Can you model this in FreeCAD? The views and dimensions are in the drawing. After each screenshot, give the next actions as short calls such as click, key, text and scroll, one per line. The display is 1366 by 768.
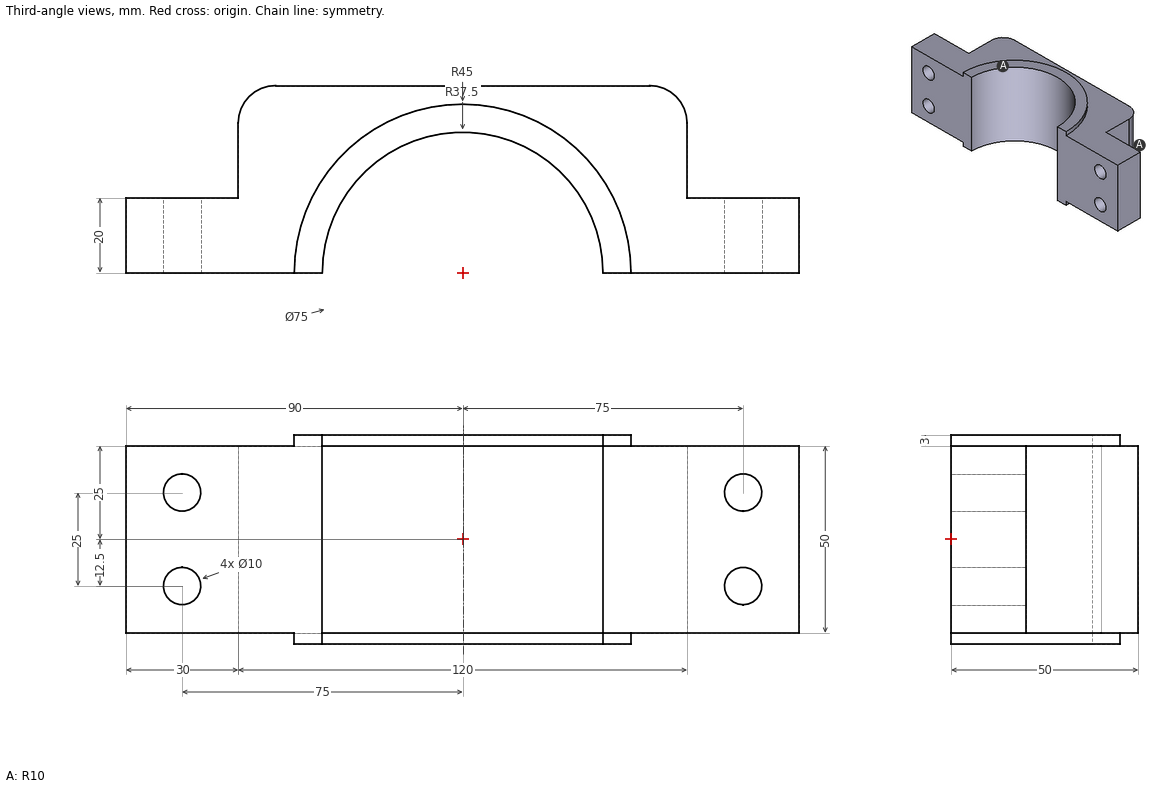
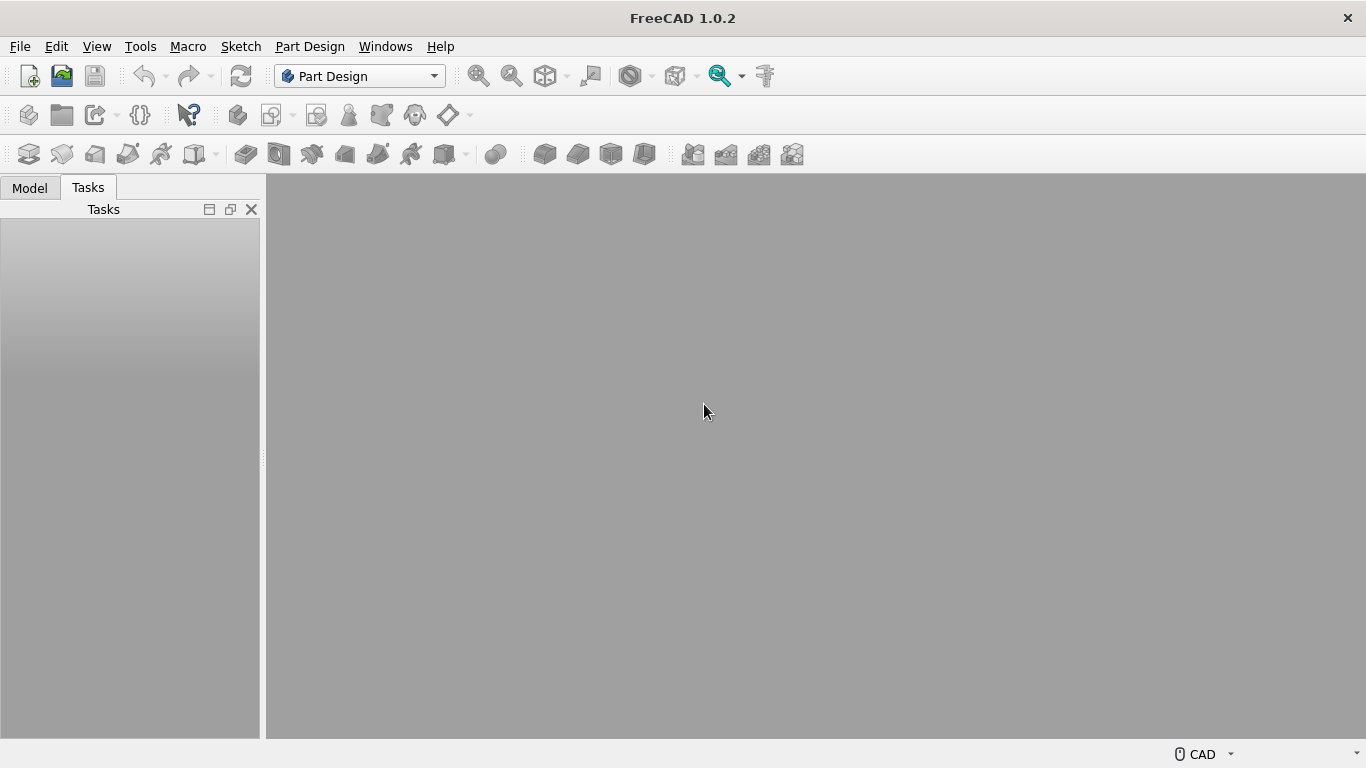
click(29, 76)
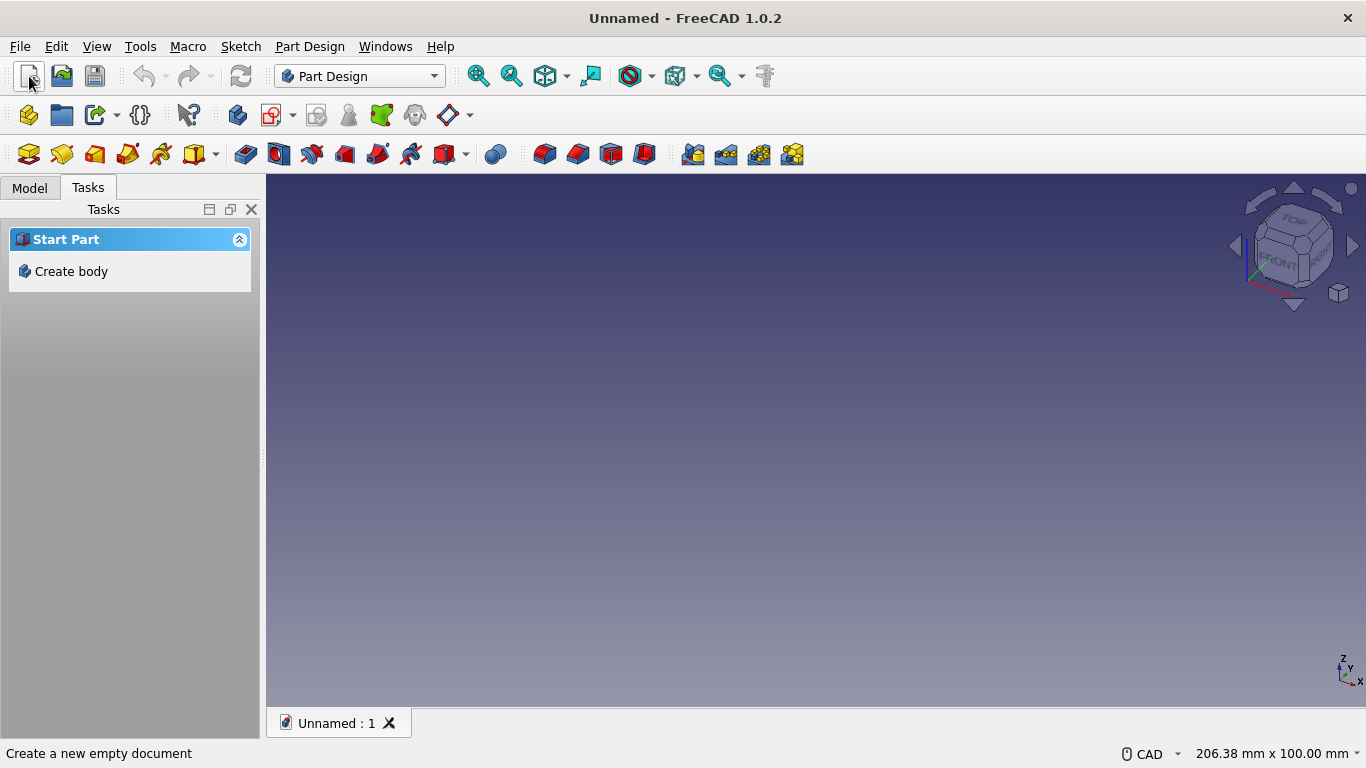
click(270, 116)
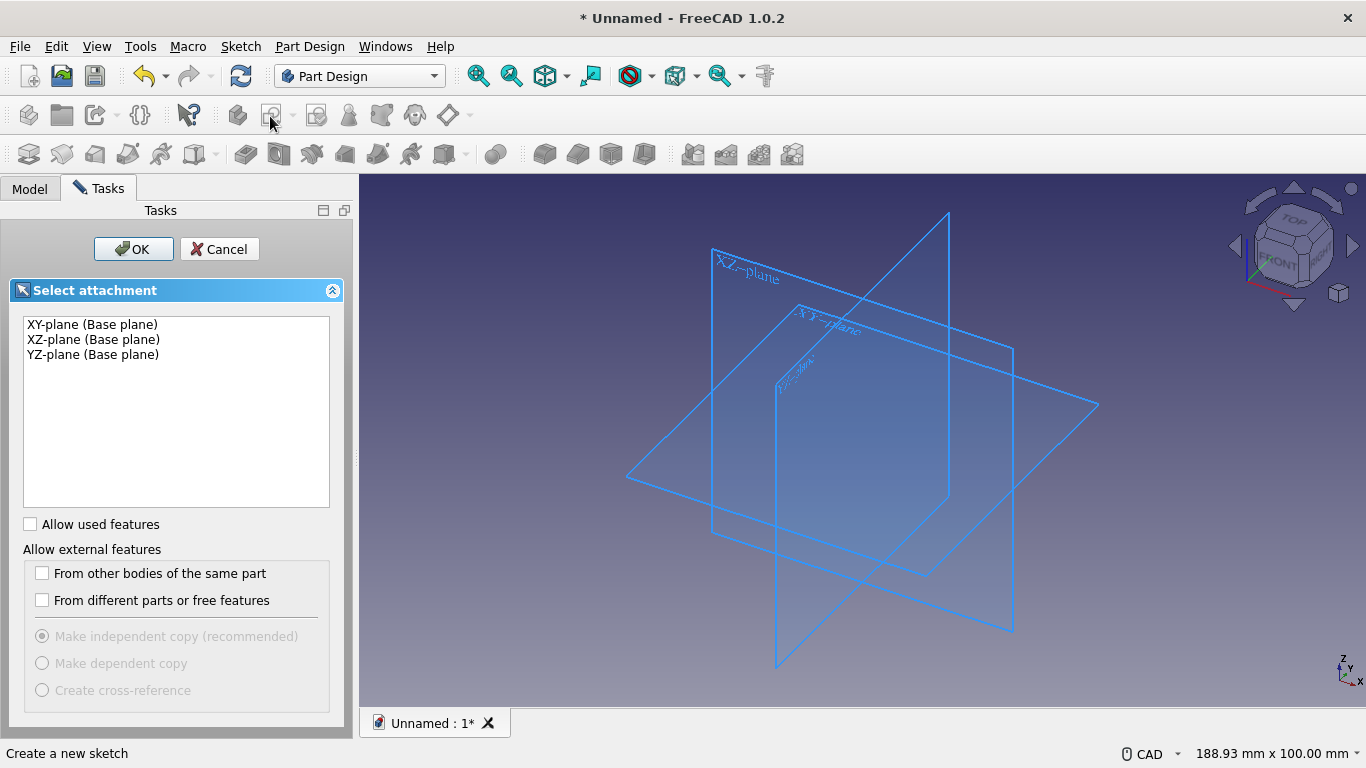
click(84, 340)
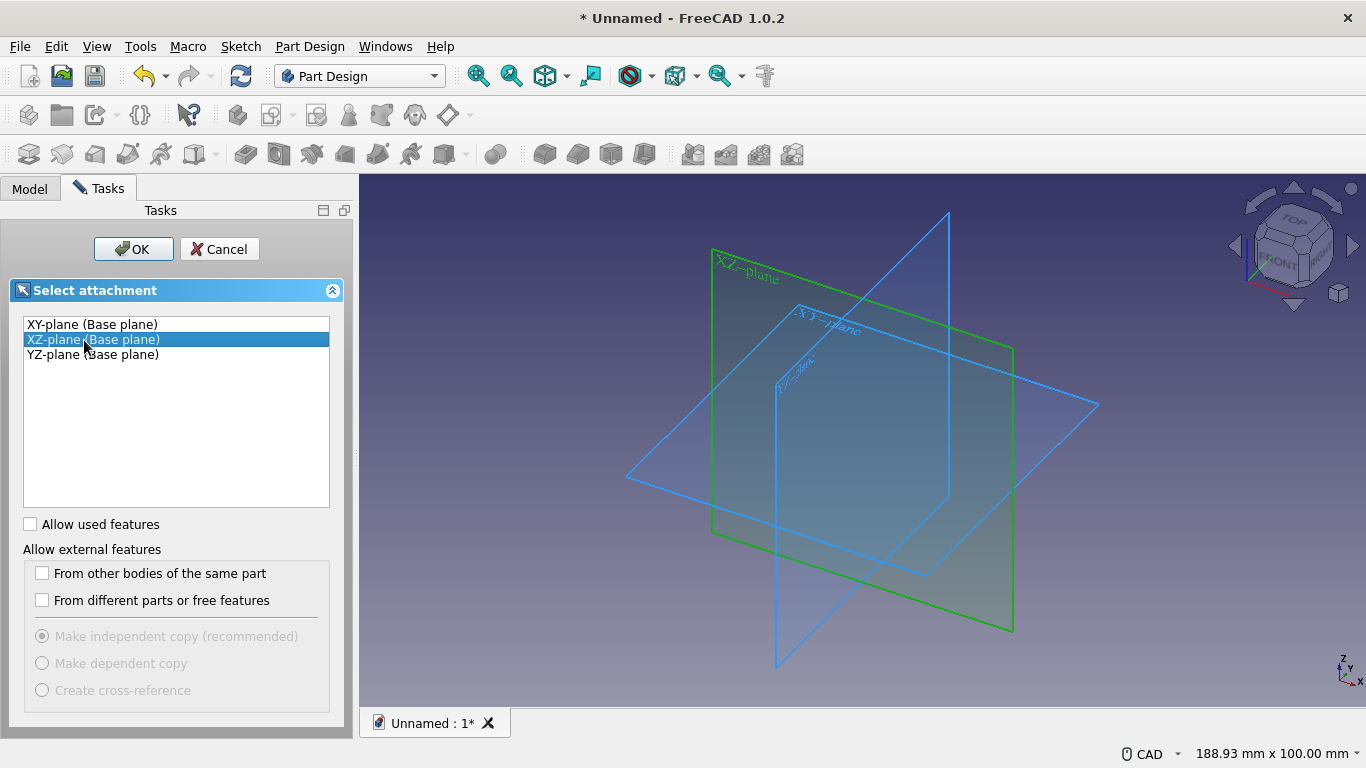
click(134, 249)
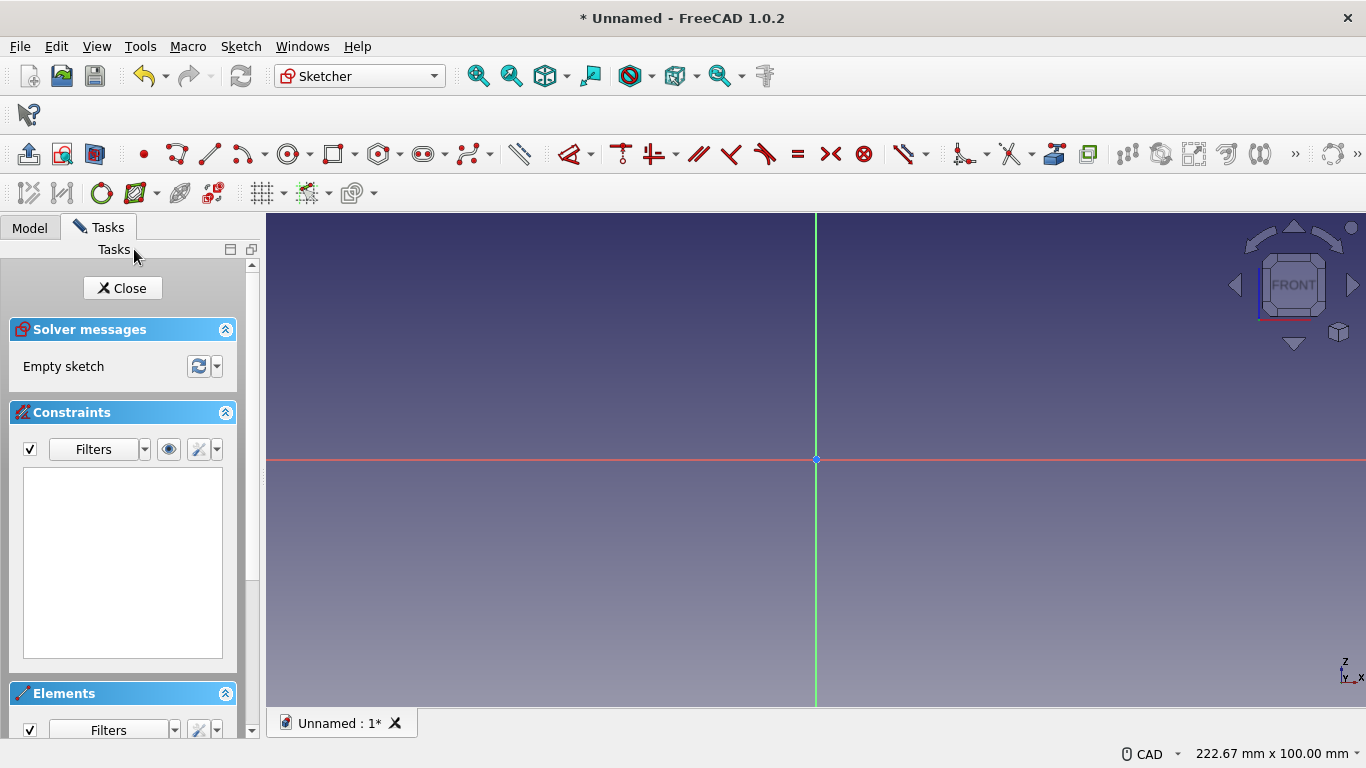
key(g)
key(v)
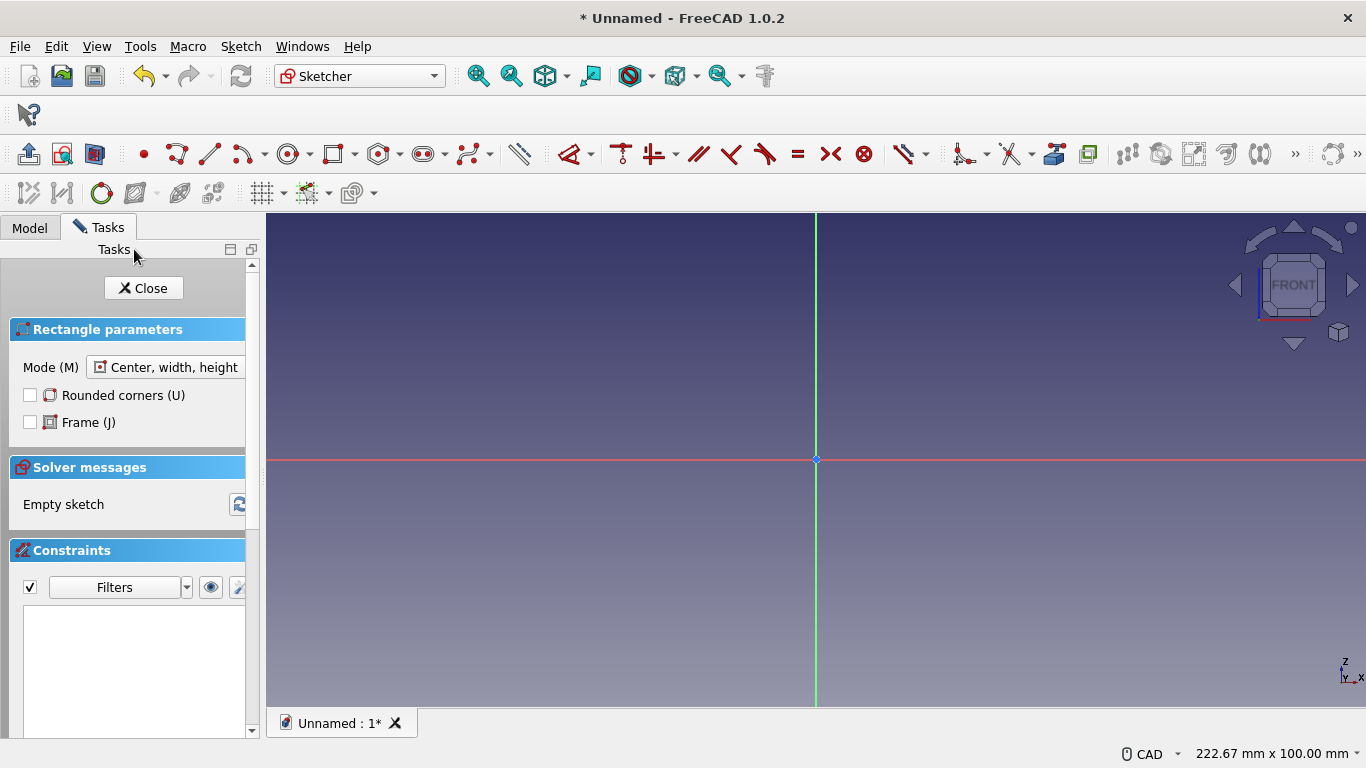
click(816, 460)
click(1112, 336)
key(Escape)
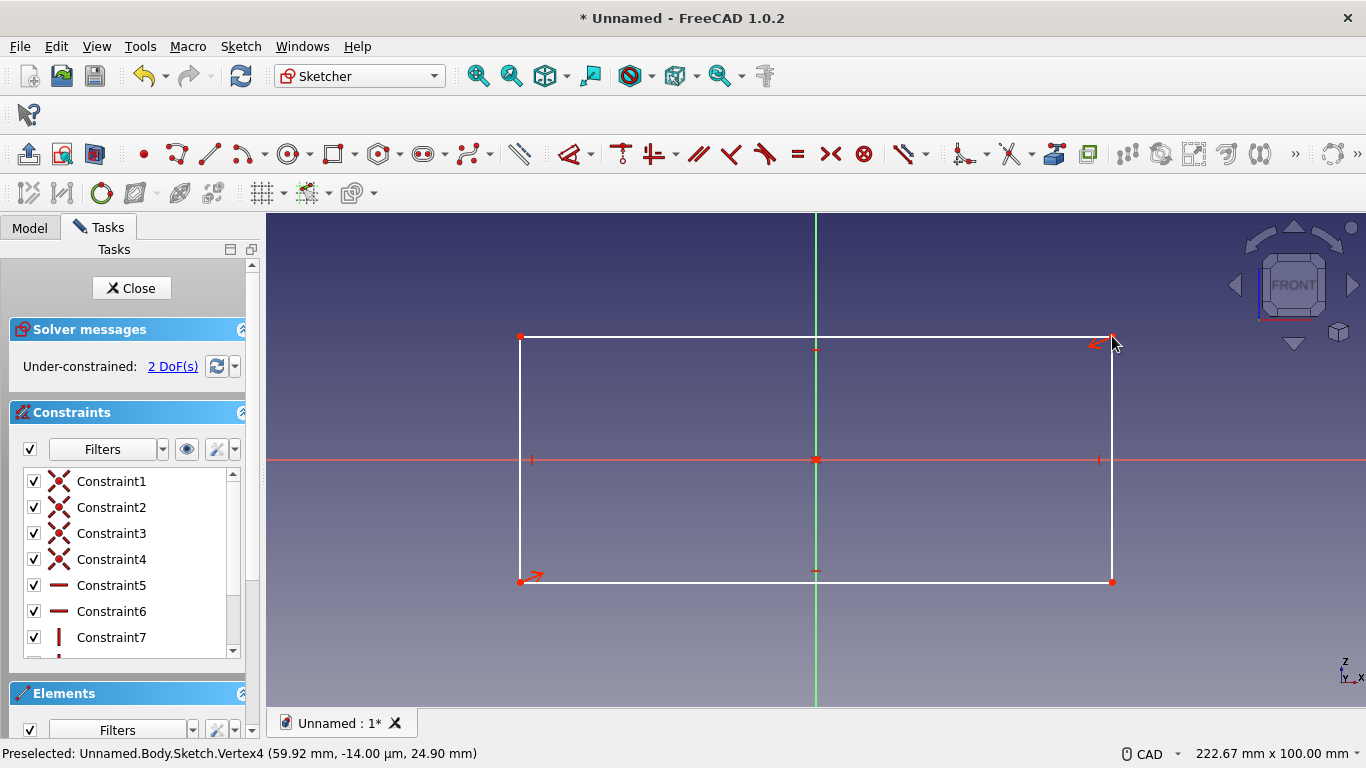
click(1112, 509)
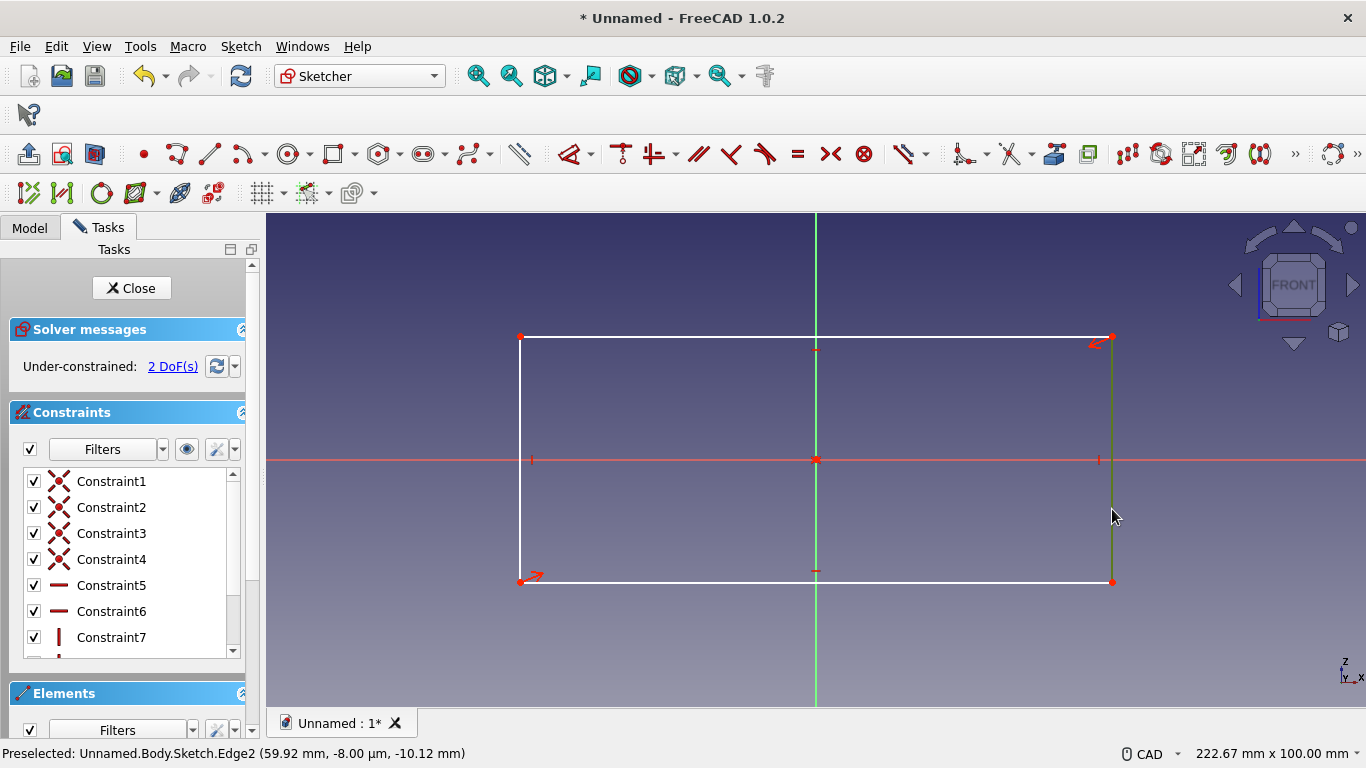
key(i)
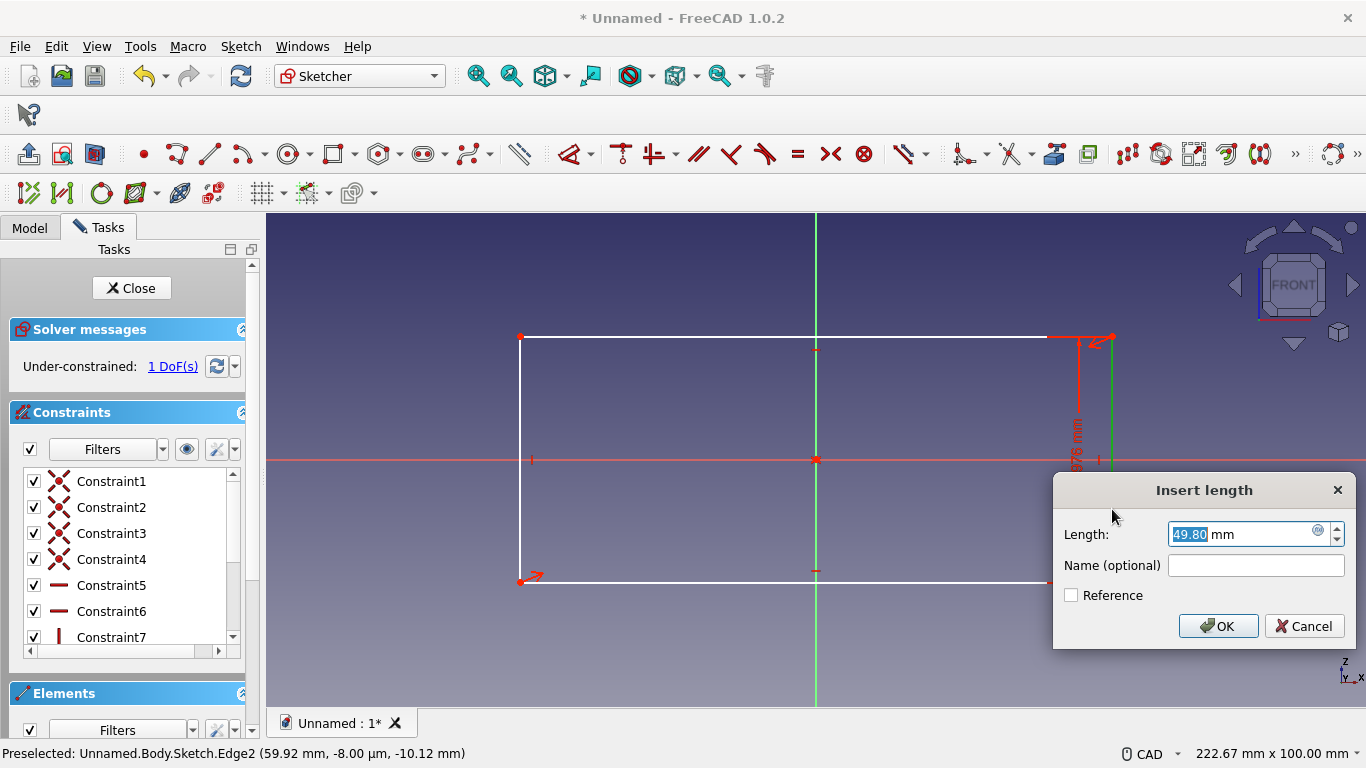
text(50)
key(Return)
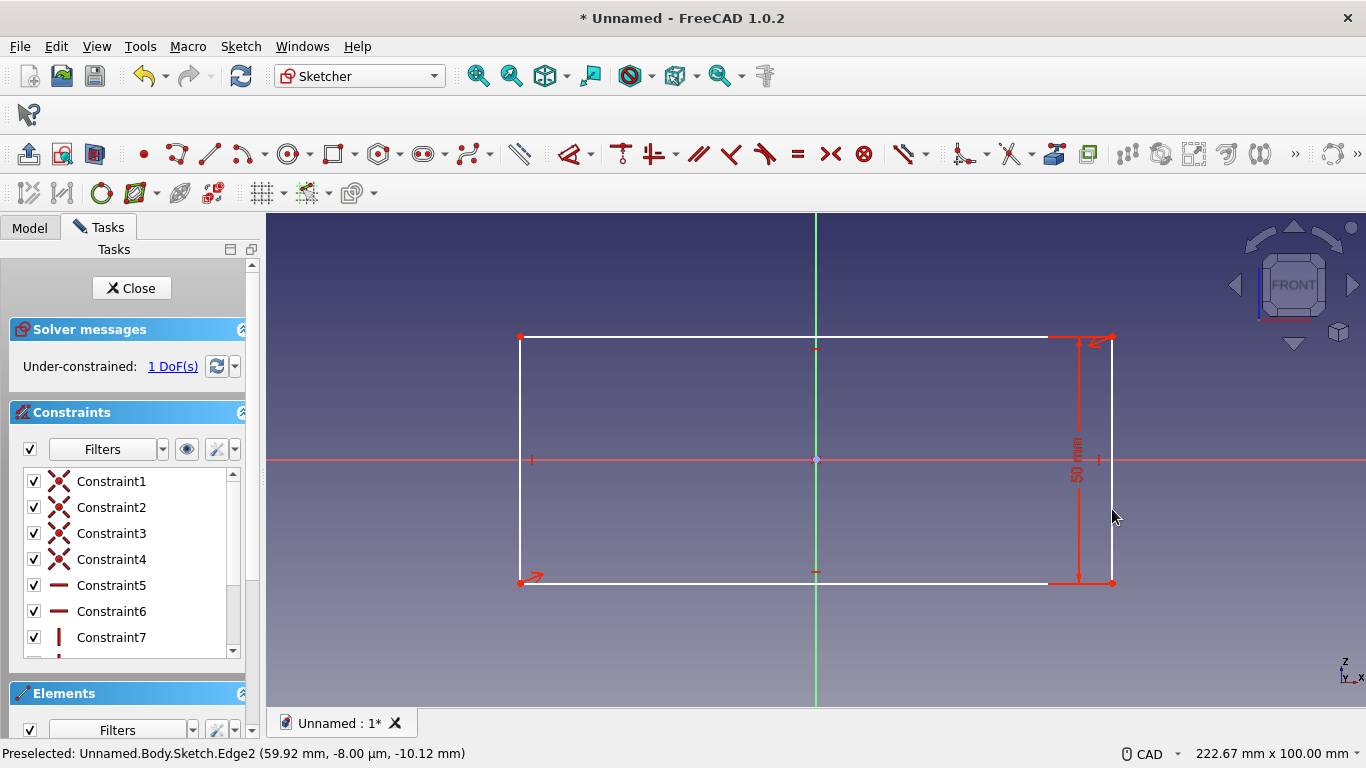
click(698, 584)